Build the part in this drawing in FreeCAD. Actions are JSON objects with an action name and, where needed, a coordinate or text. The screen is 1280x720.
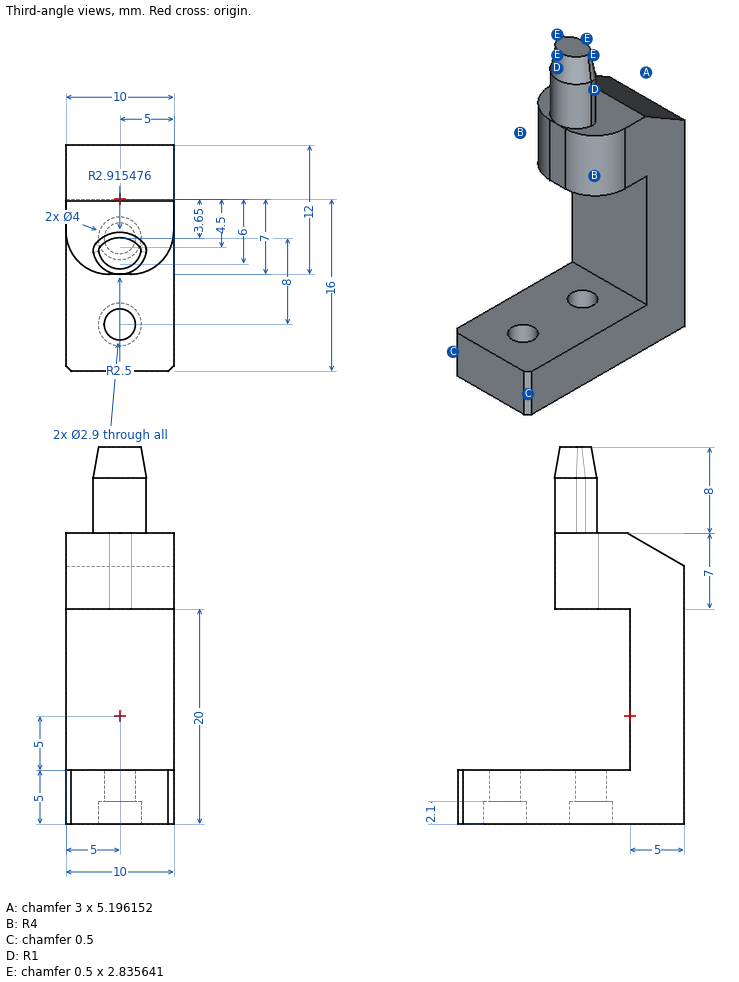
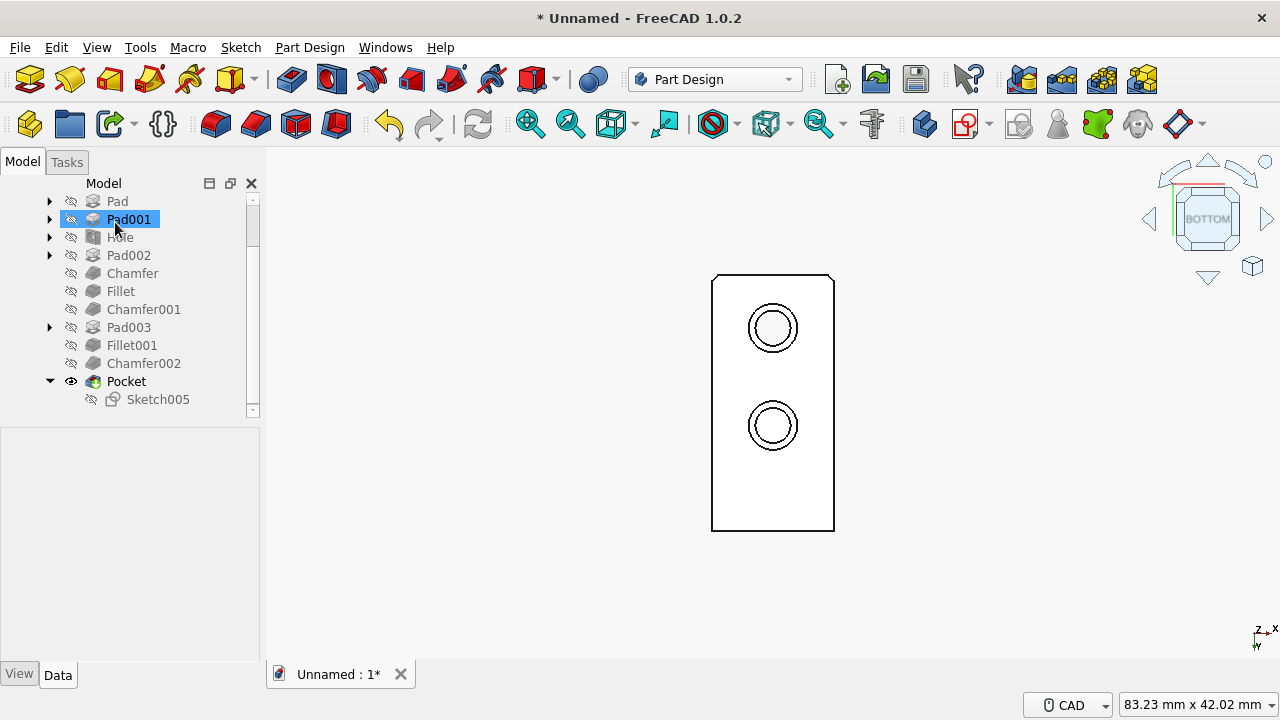
{"action": "key", "text": "0"}